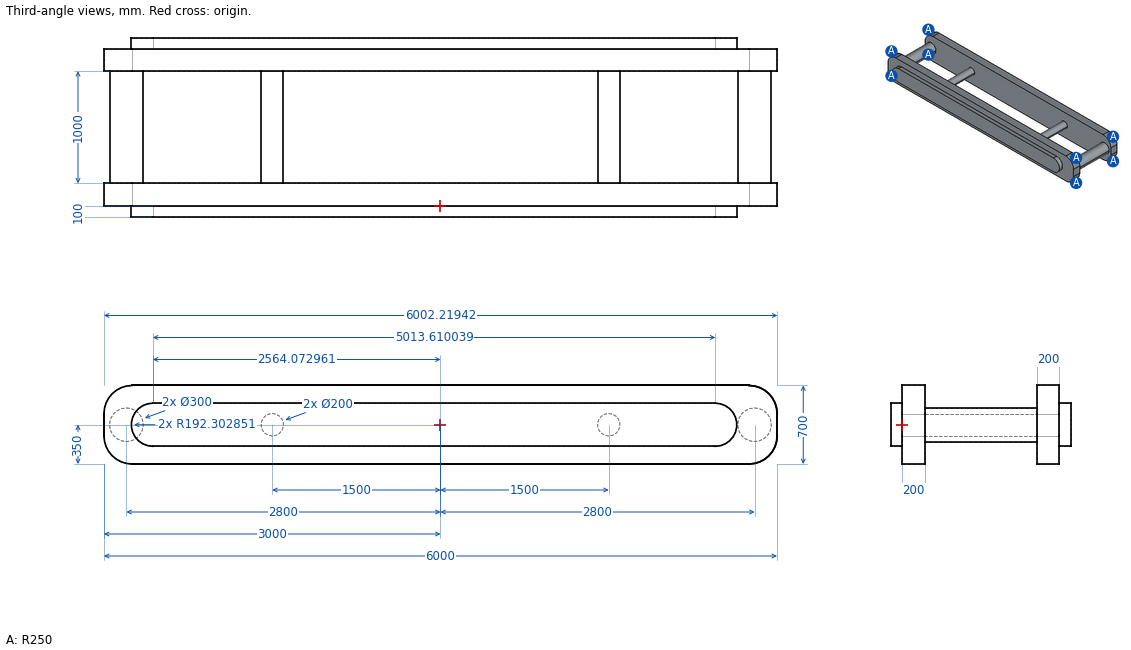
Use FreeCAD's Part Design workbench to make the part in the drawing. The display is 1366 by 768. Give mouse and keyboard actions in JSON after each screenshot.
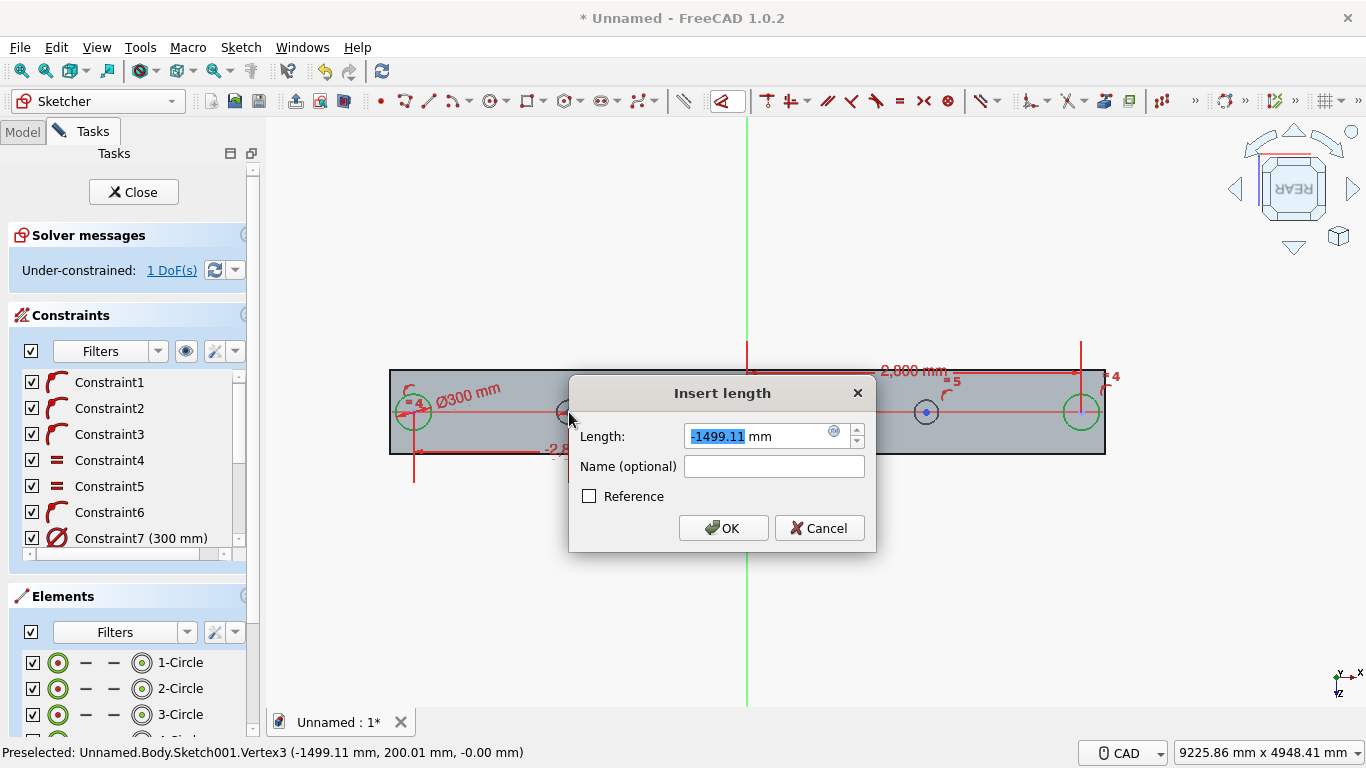
{"action": "type", "text": "-1500"}
{"action": "key", "text": "Return"}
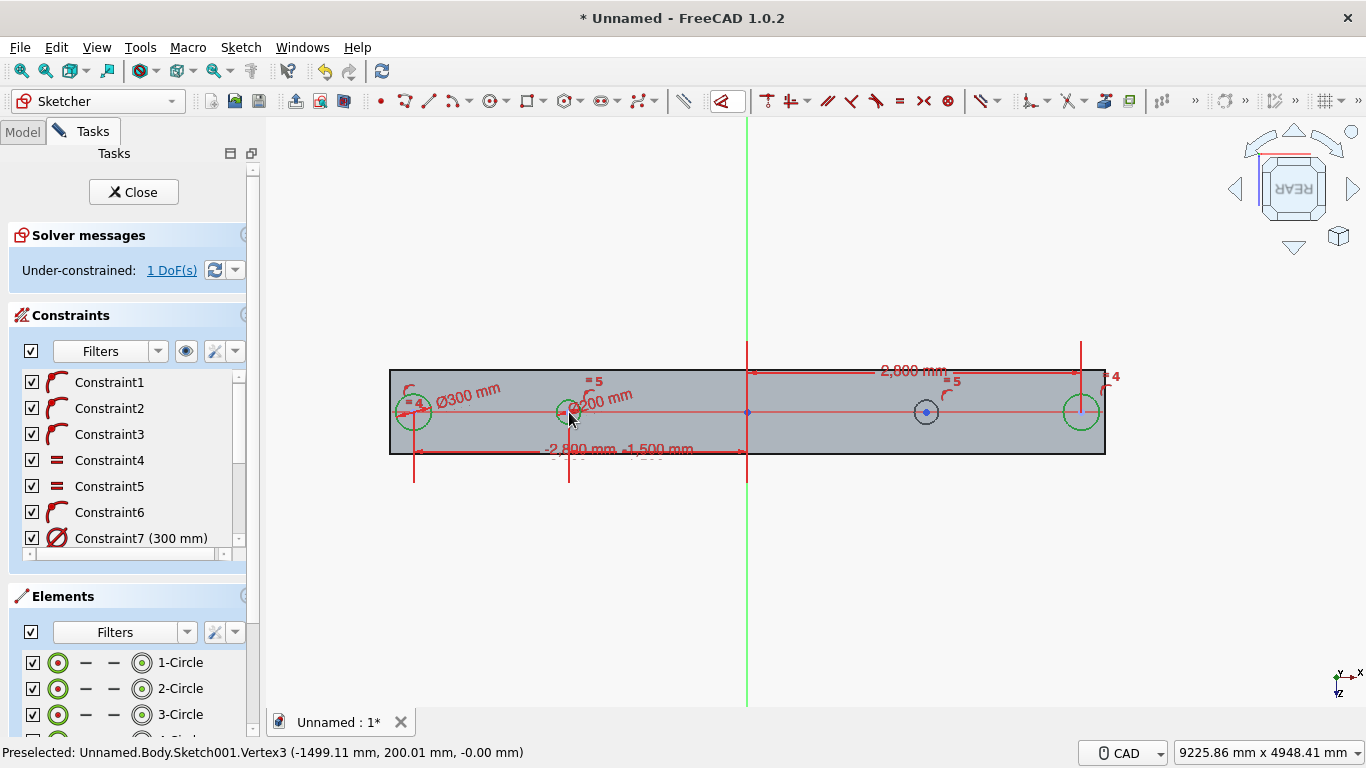
{"action": "left_click", "coordinate": [926, 412]}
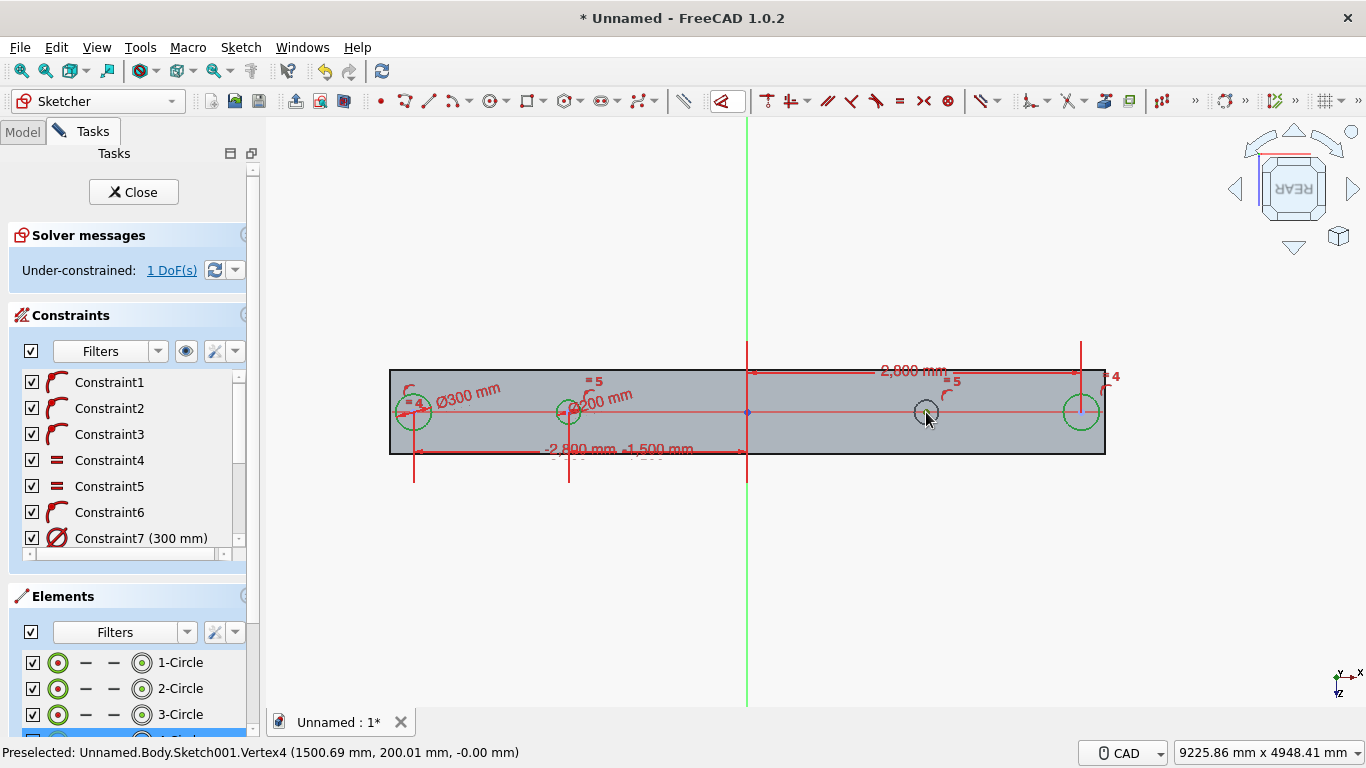
{"action": "key", "text": "l"}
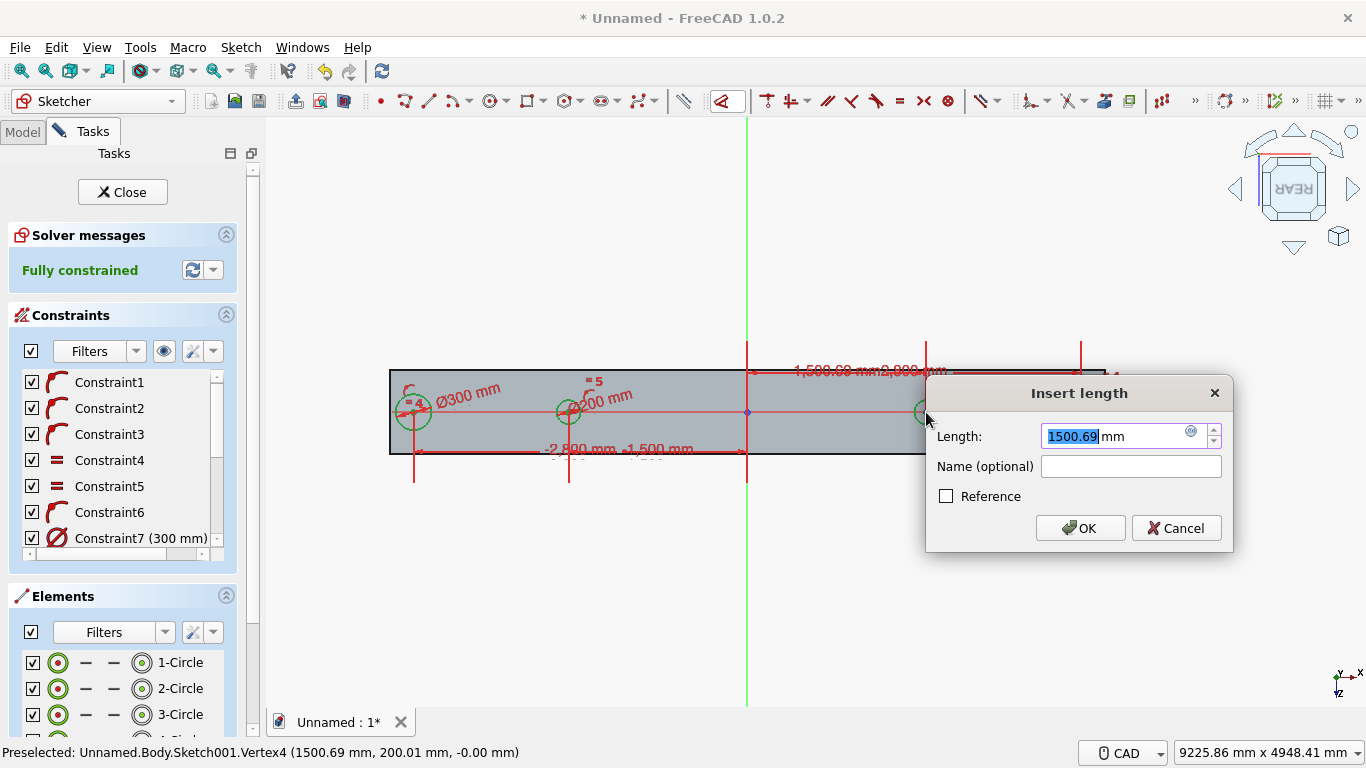
{"action": "type", "text": "1500"}
{"action": "key", "text": "Return"}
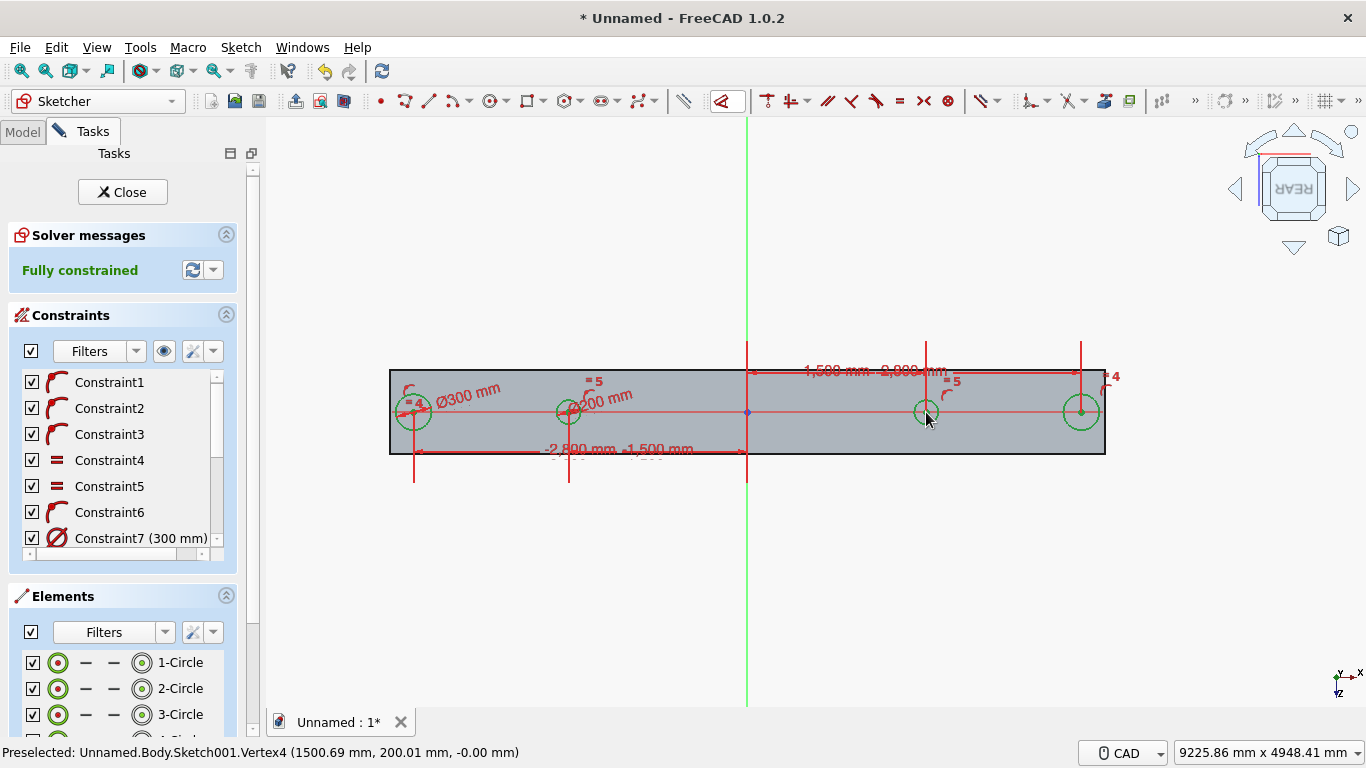
{"action": "left_click", "coordinate": [123, 192]}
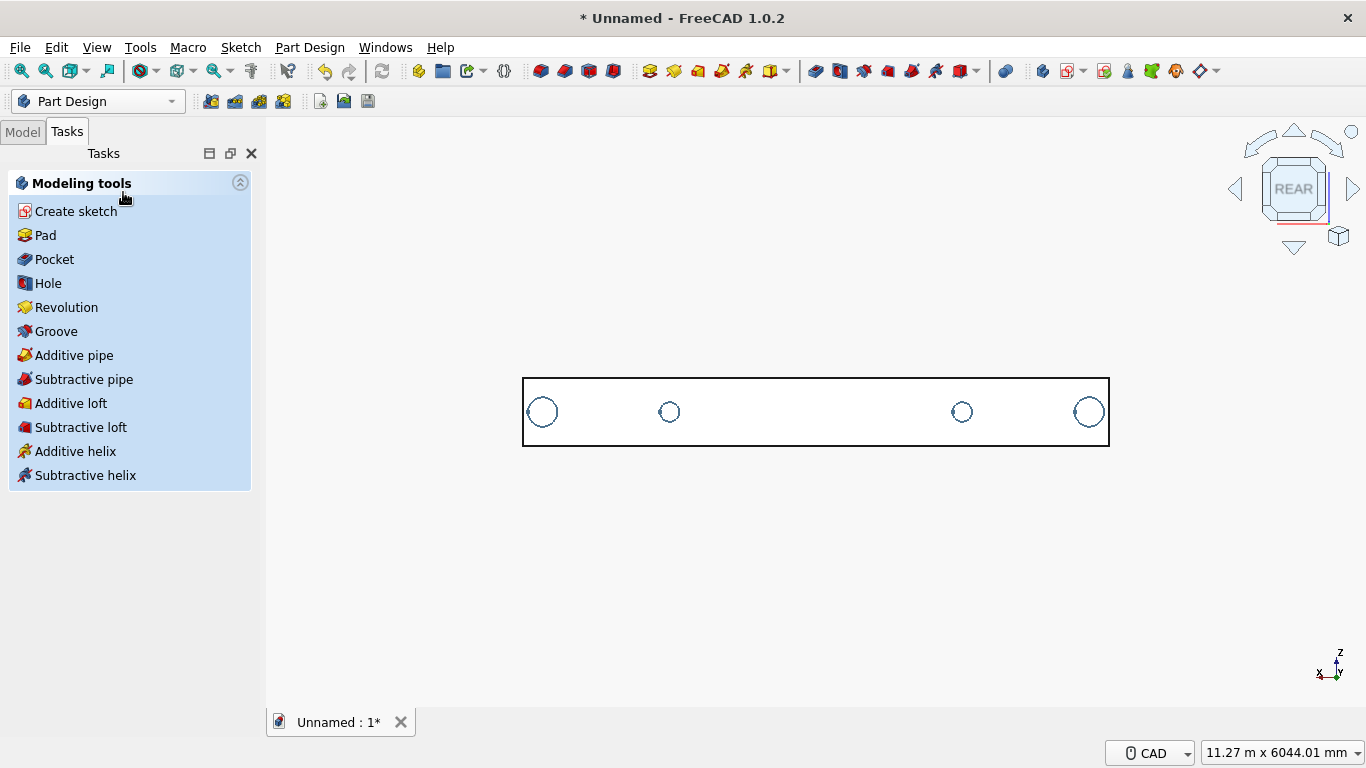
{"action": "left_click", "coordinate": [650, 72]}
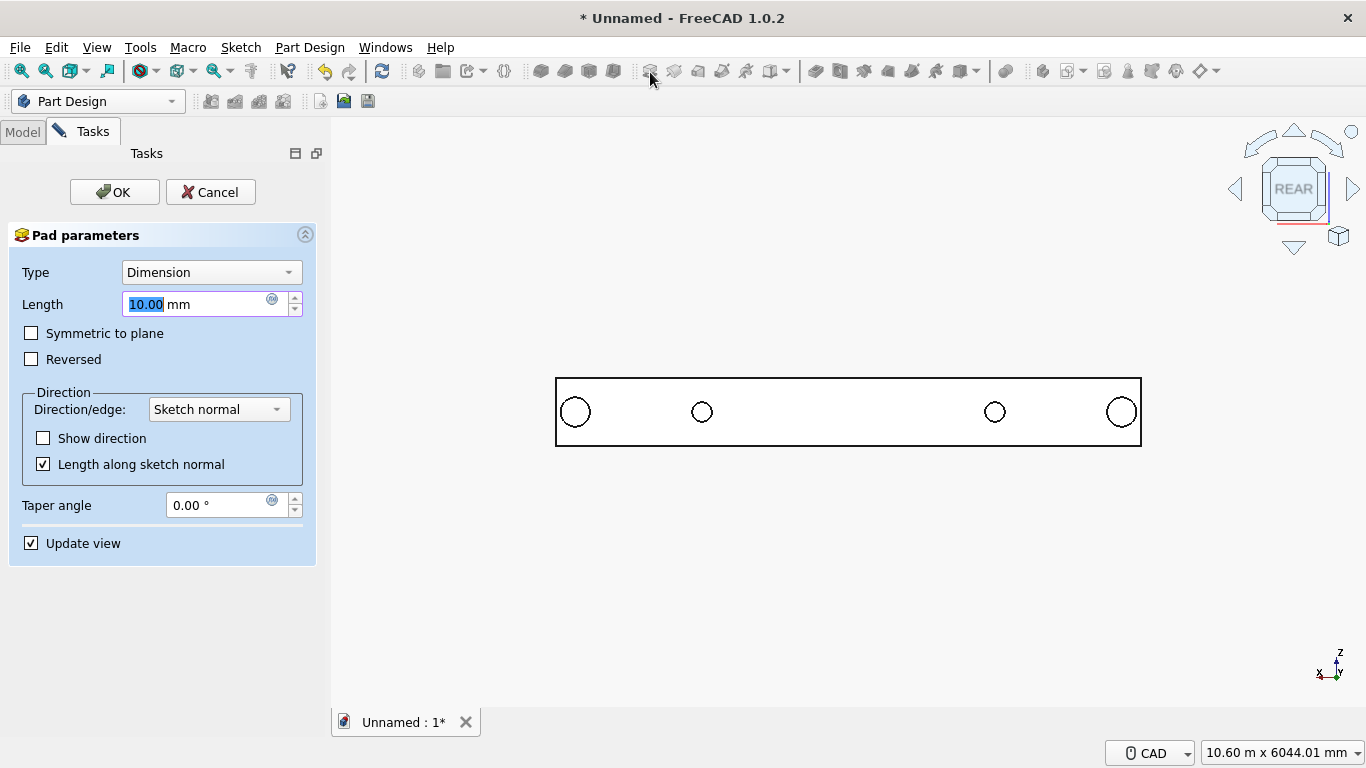
{"action": "type", "text": "1000"}
{"action": "key", "text": "Tab"}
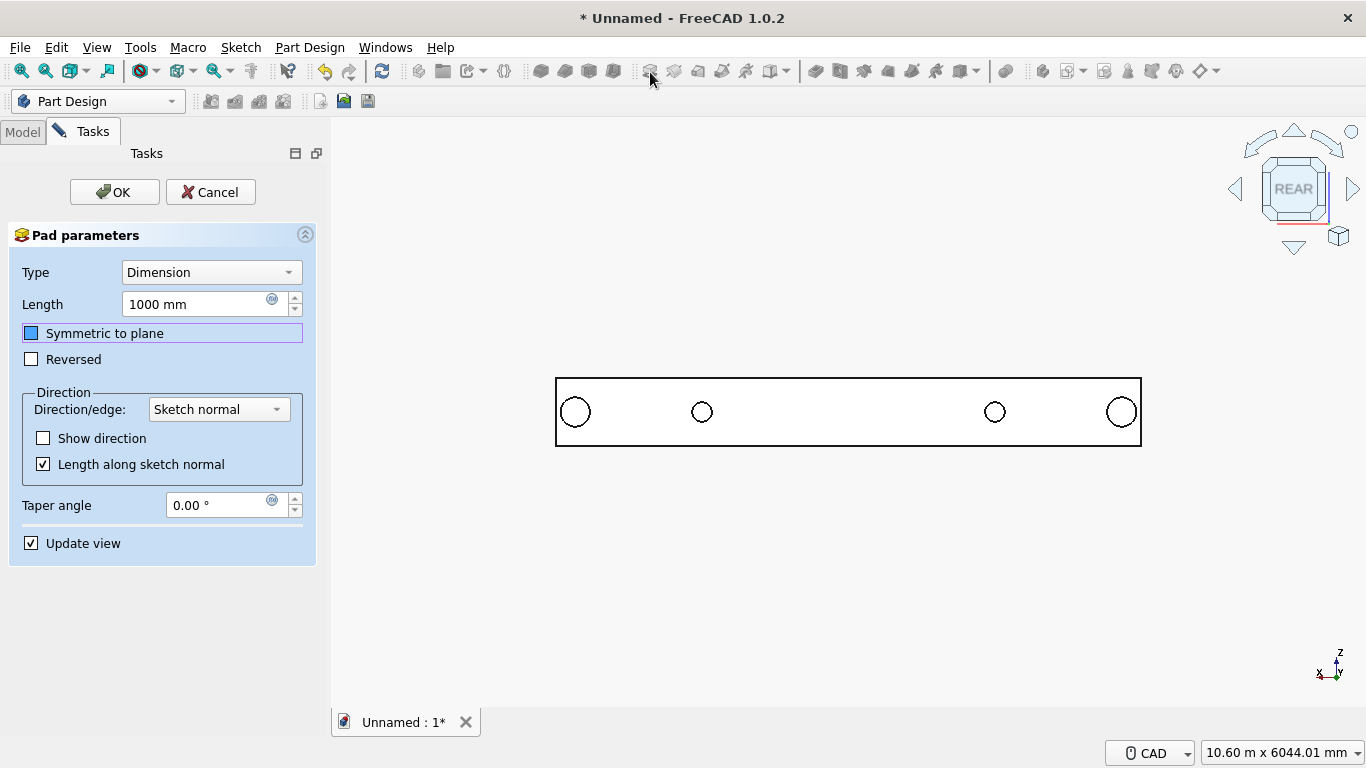
{"action": "left_click", "coordinate": [115, 192]}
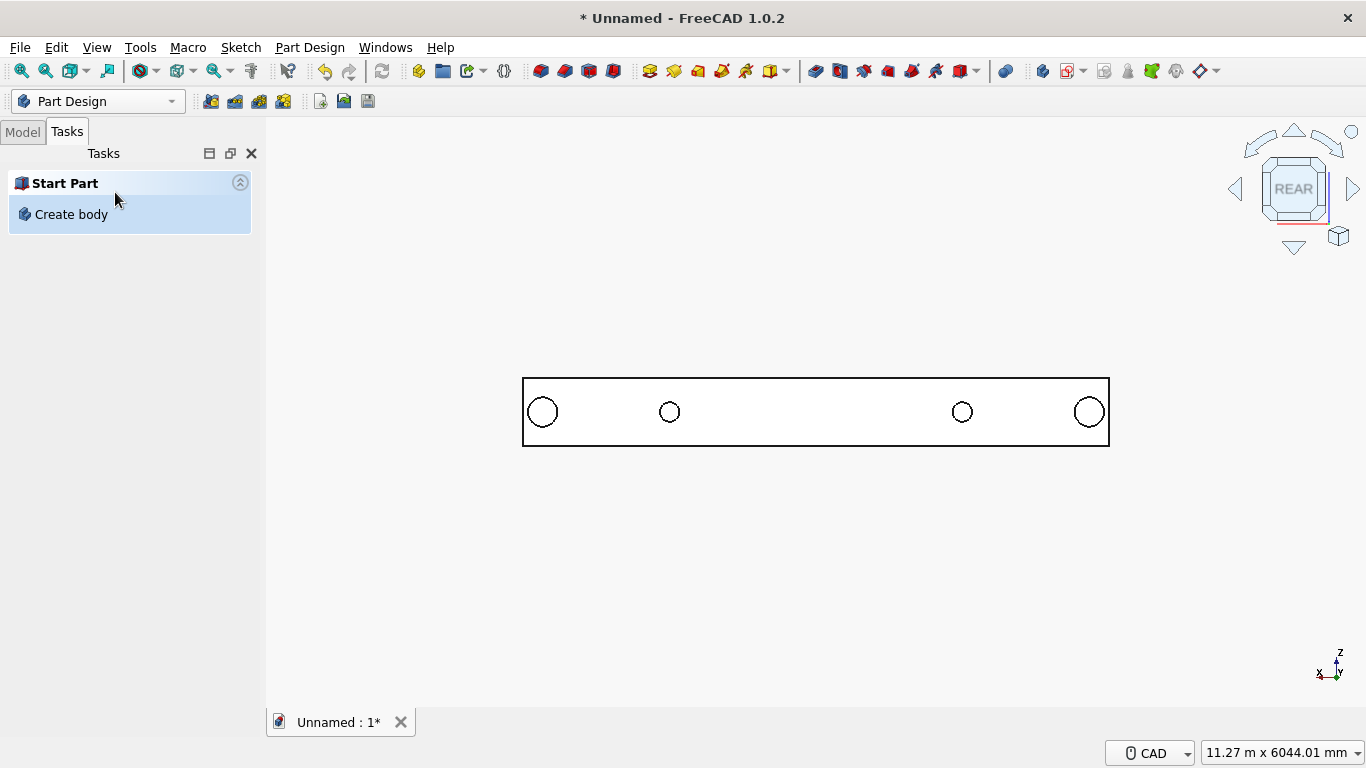
{"action": "left_click", "coordinate": [543, 411]}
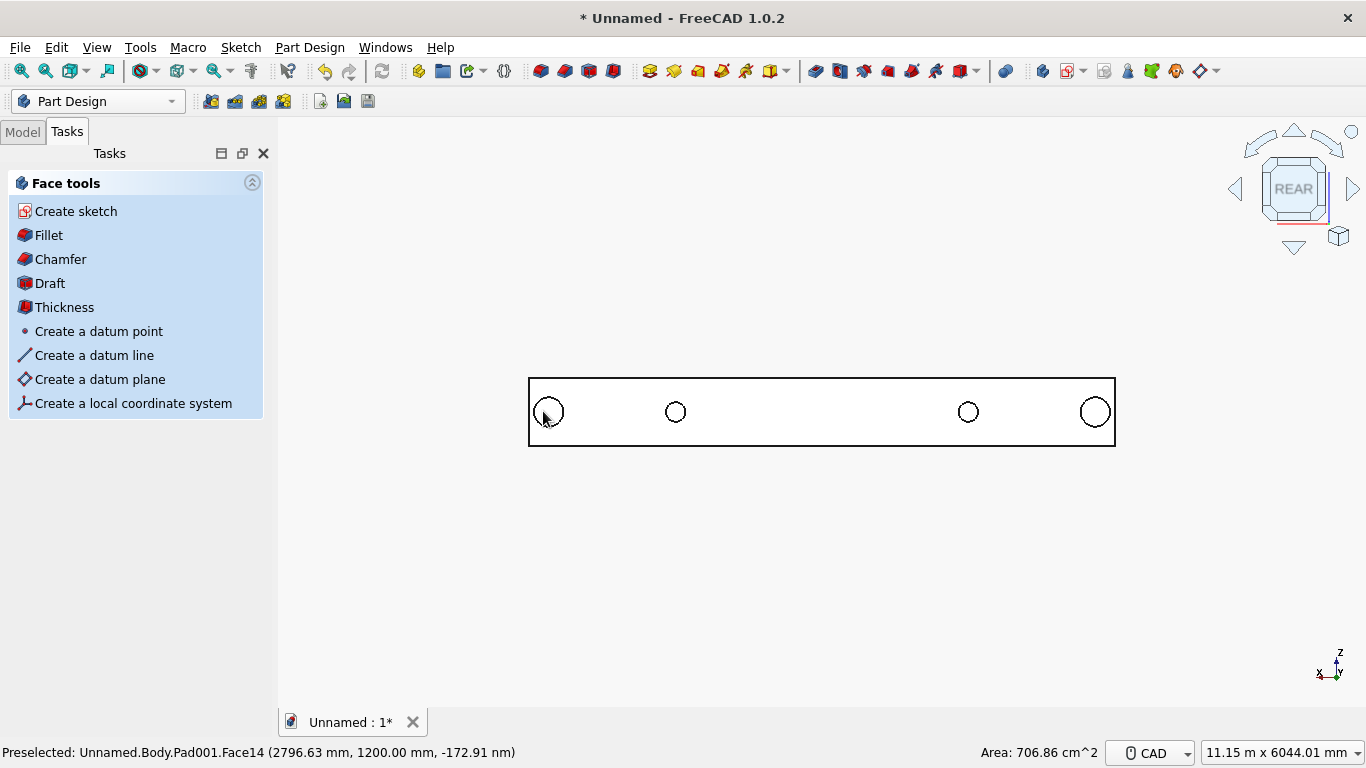
{"action": "left_click", "coordinate": [1068, 72]}